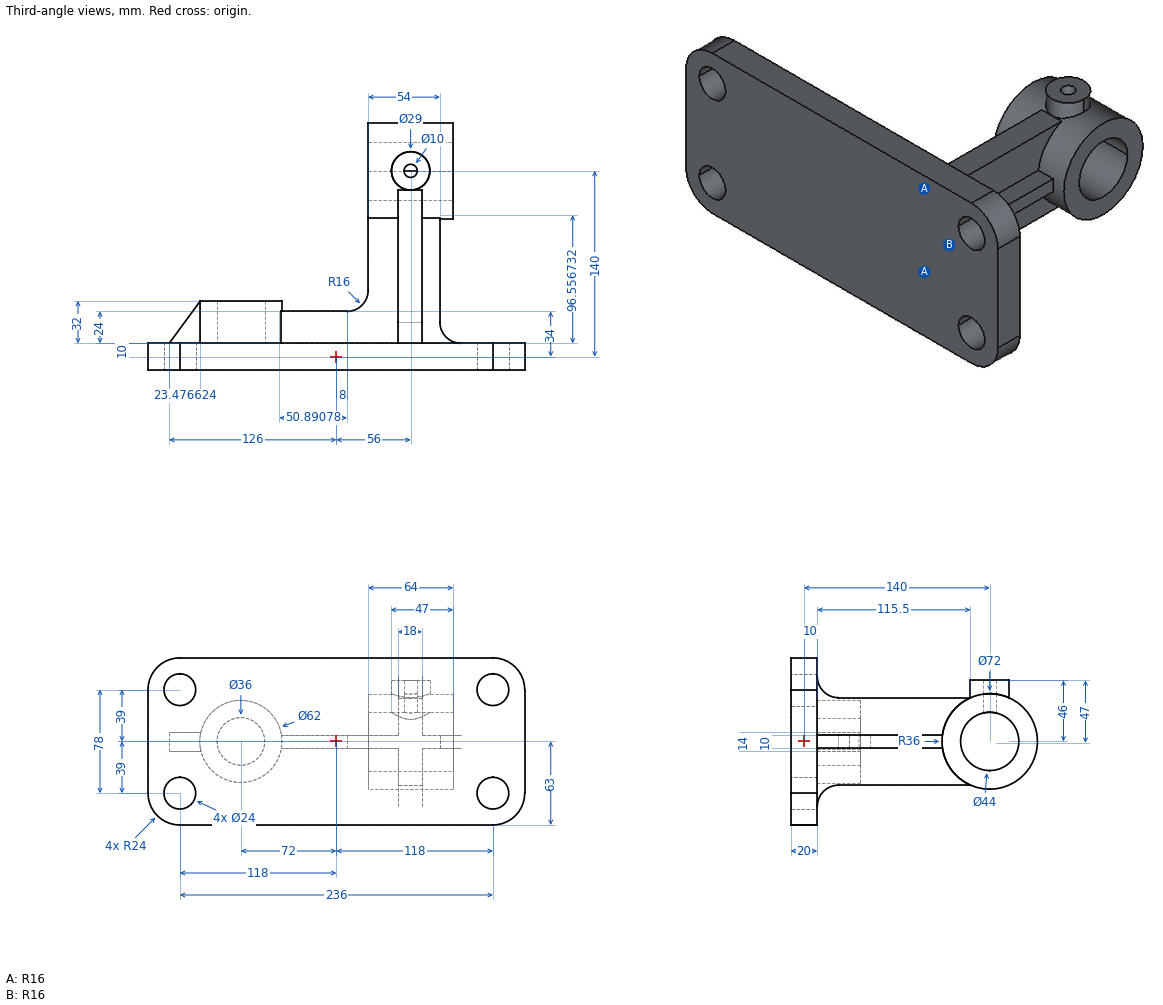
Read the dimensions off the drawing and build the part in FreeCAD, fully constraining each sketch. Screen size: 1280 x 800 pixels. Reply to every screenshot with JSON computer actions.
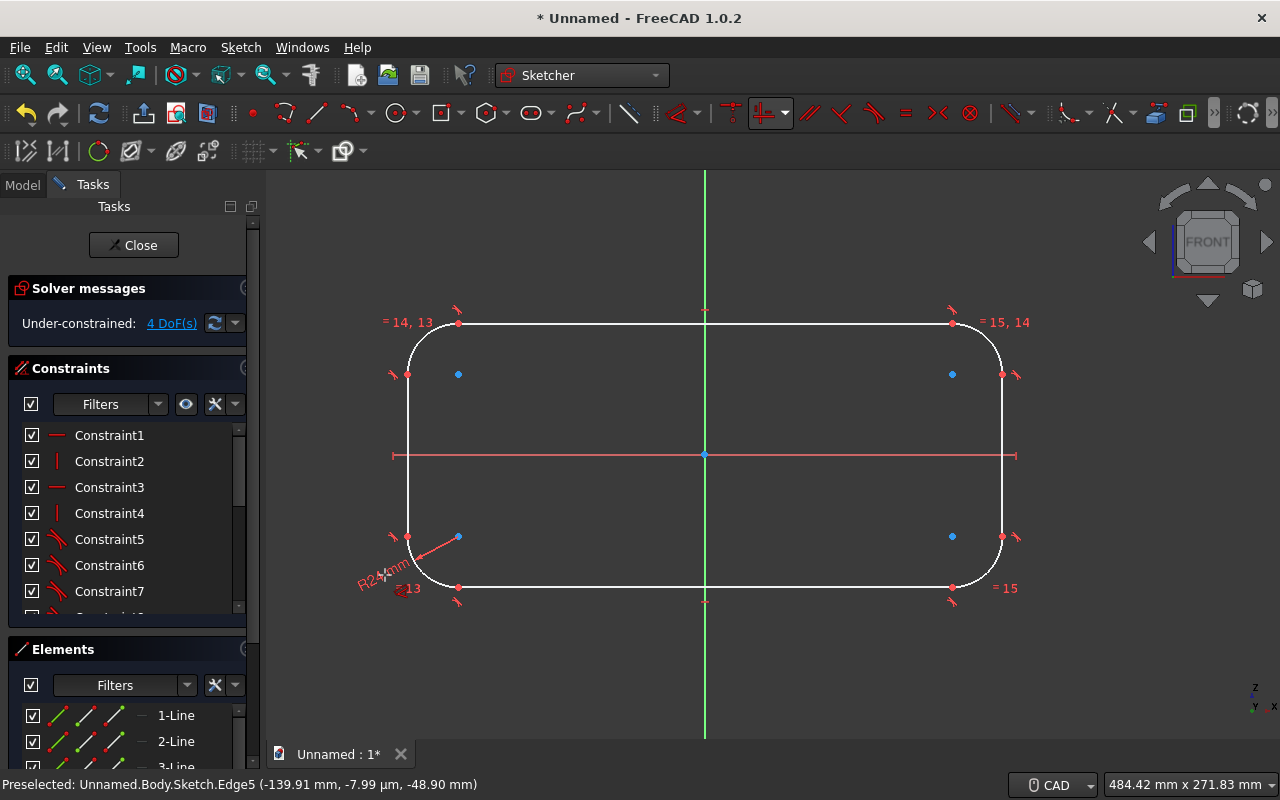
{"action": "left_click", "coordinate": [408, 488]}
{"action": "left_click", "coordinate": [374, 418]}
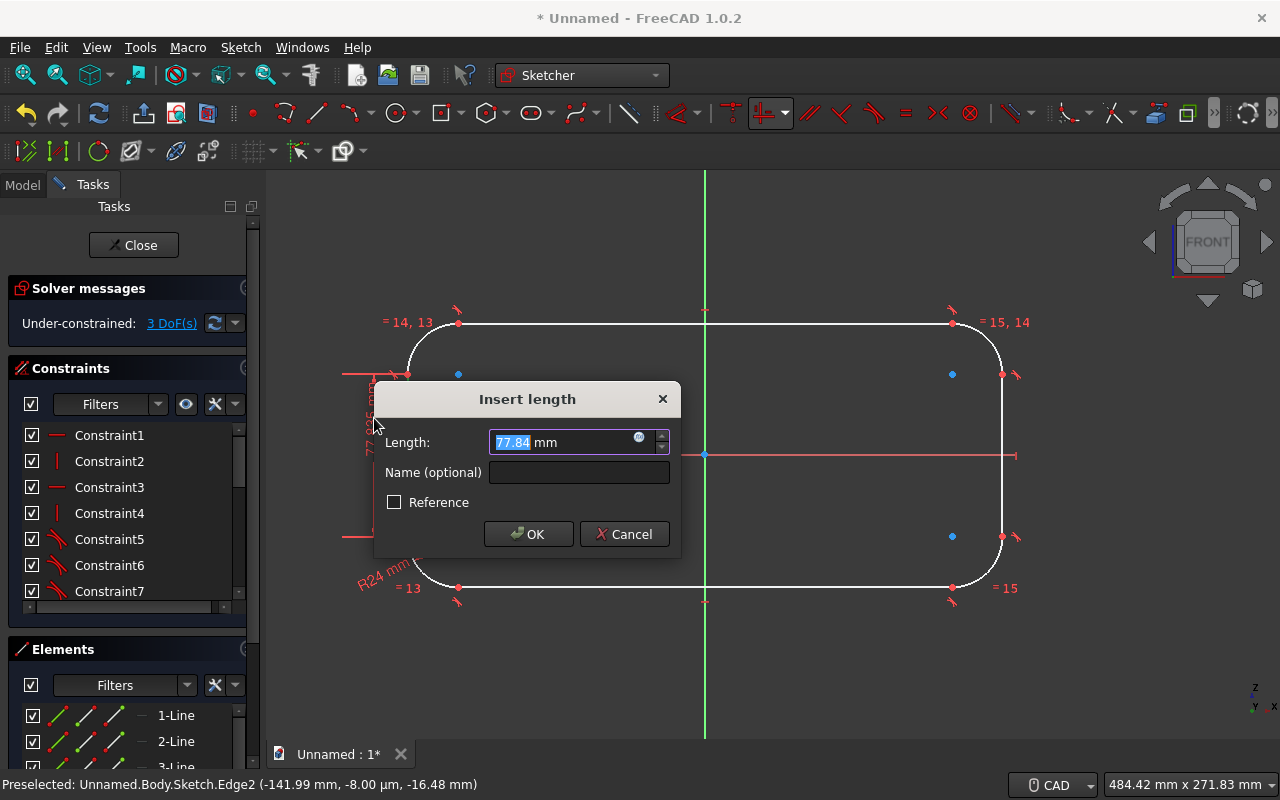
{"action": "type", "text": "78"}
{"action": "key", "text": "Return"}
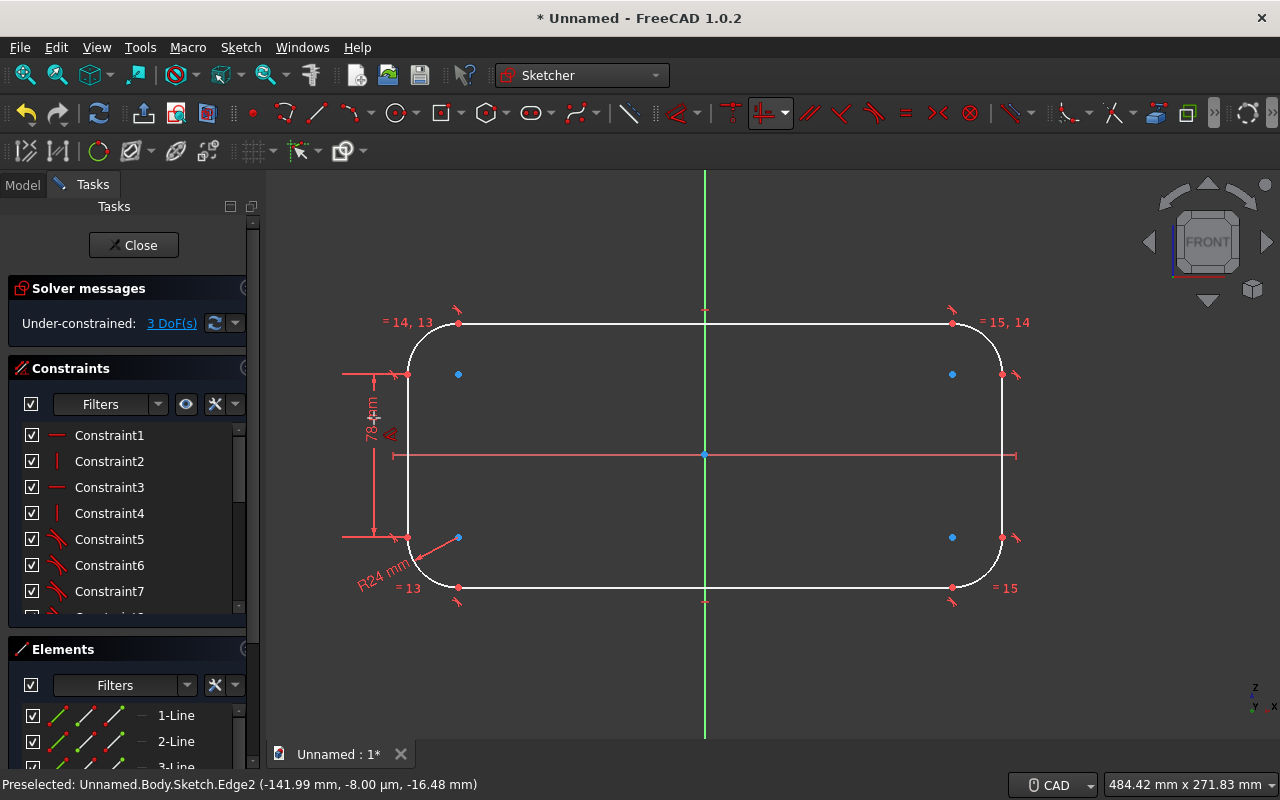
{"action": "left_click", "coordinate": [804, 588]}
{"action": "left_click", "coordinate": [591, 622]}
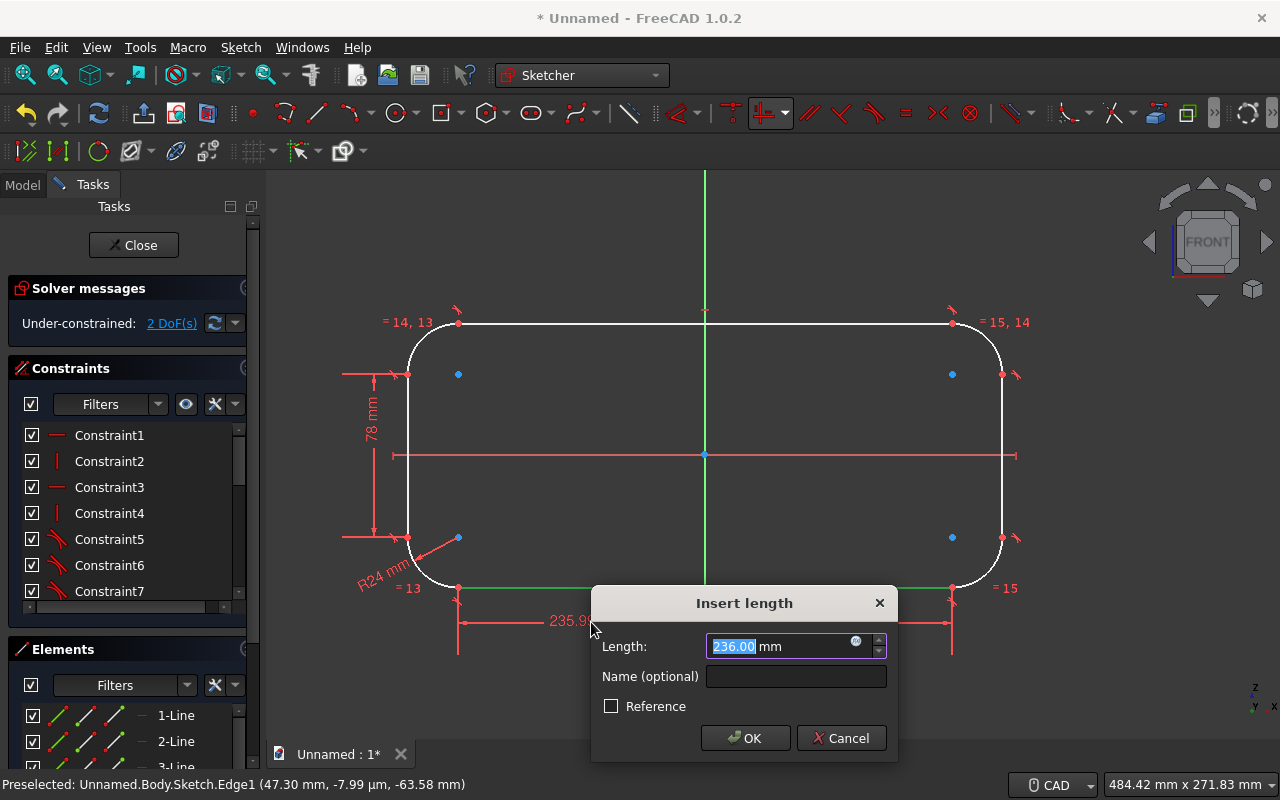
{"action": "type", "text": "236"}
{"action": "key", "text": "Return"}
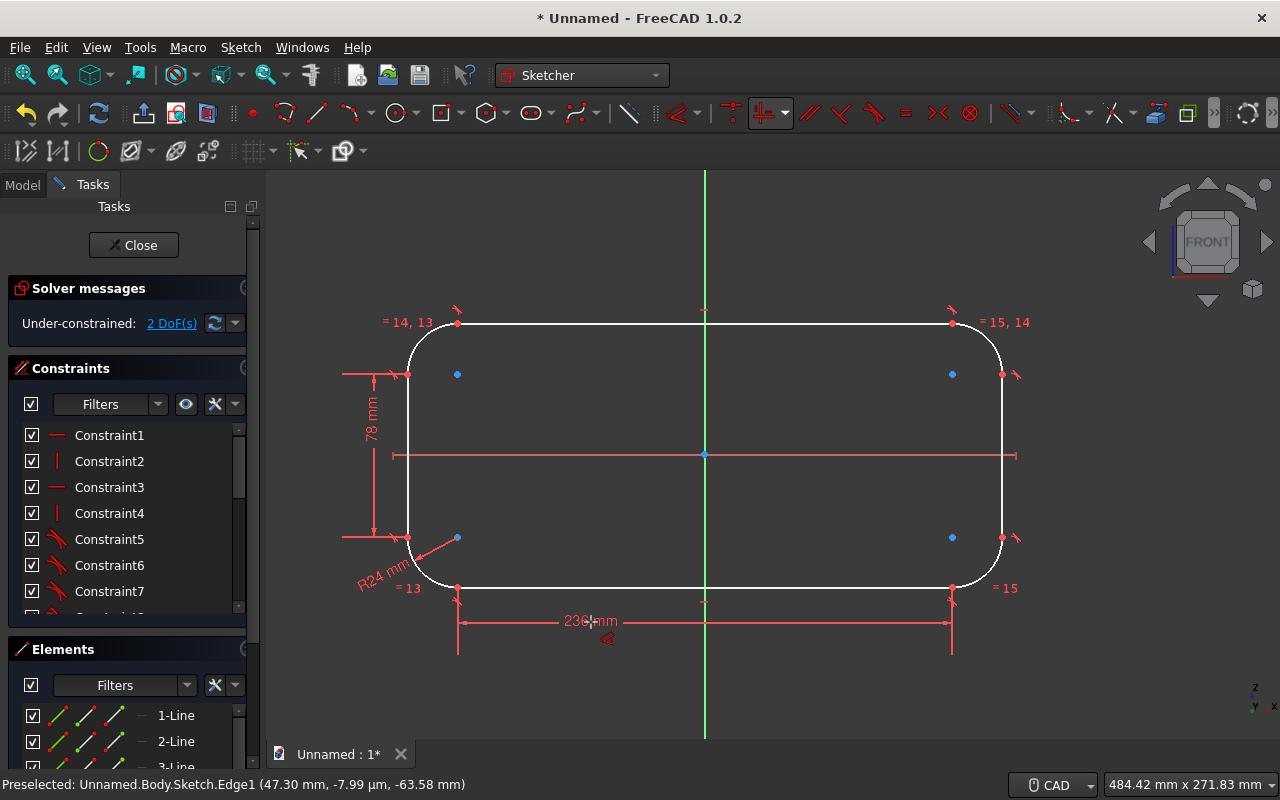
{"action": "left_click", "coordinate": [952, 588]}
{"action": "left_click", "coordinate": [986, 521]}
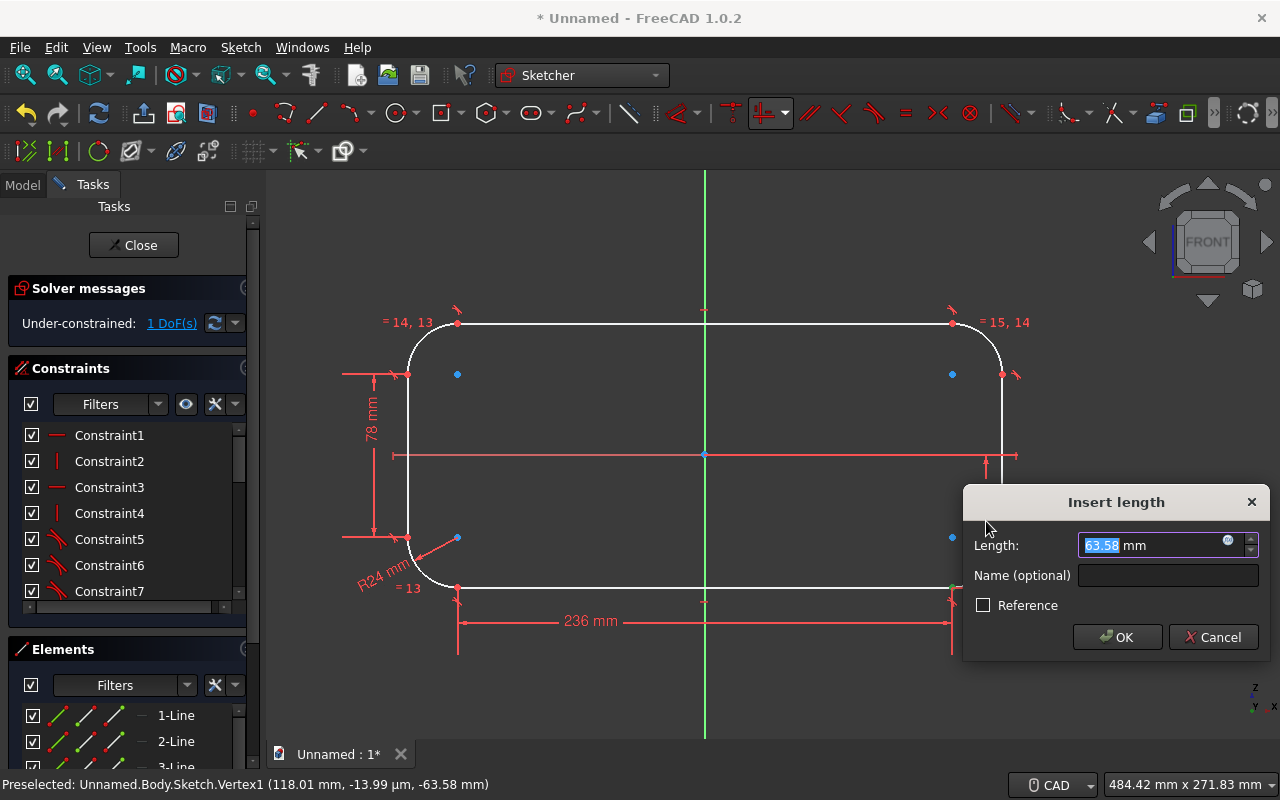
{"action": "type", "text": "63"}
{"action": "key", "text": "Return"}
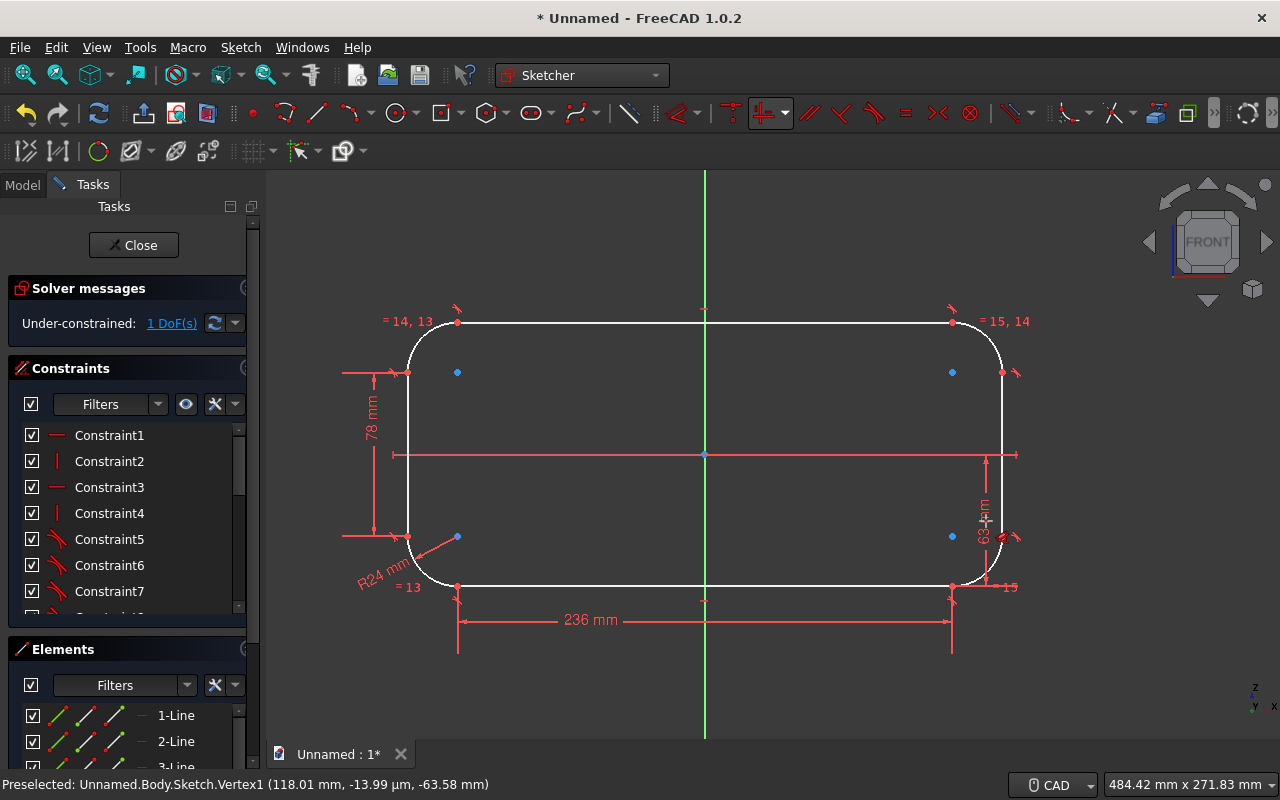
{"action": "left_click", "coordinate": [952, 586]}
{"action": "left_click", "coordinate": [828, 620]}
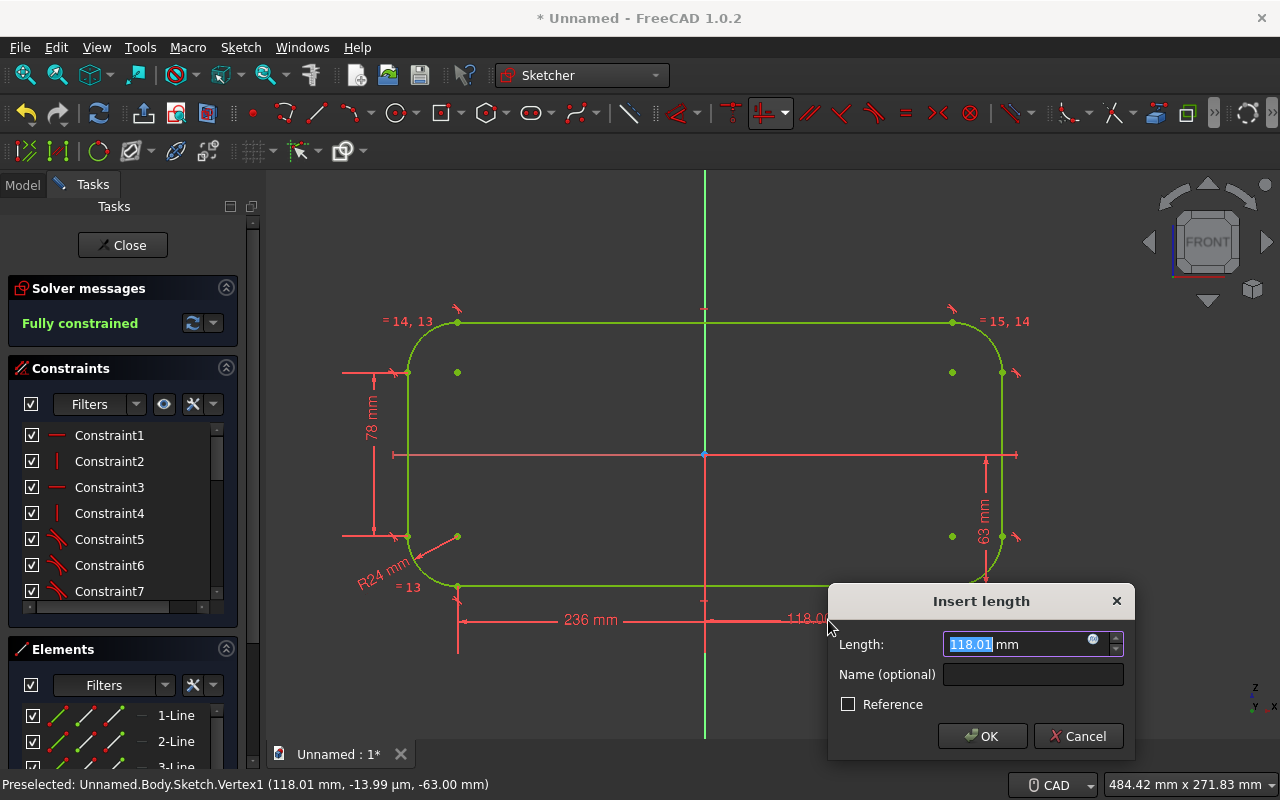
{"action": "type", "text": "118"}
{"action": "key", "text": "Return"}
{"action": "key", "text": "Escape"}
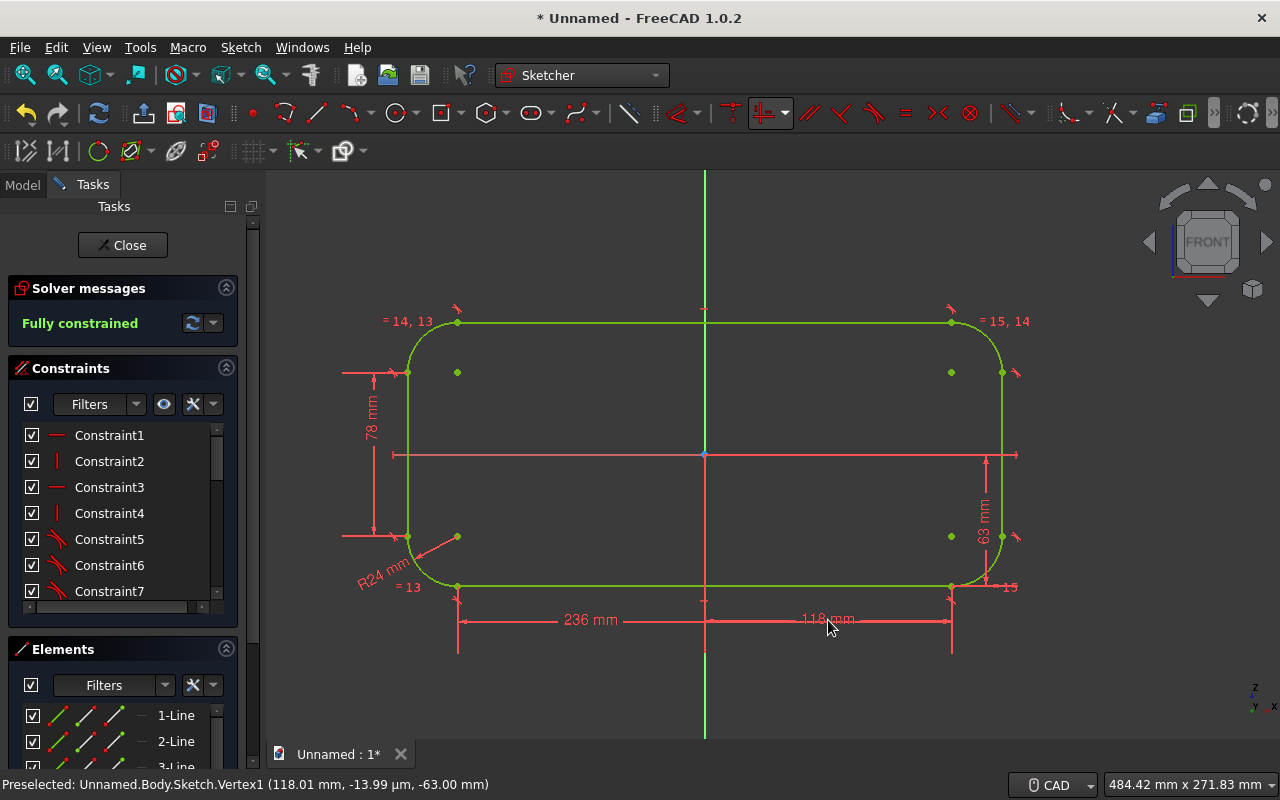
{"action": "left_click", "coordinate": [123, 245]}